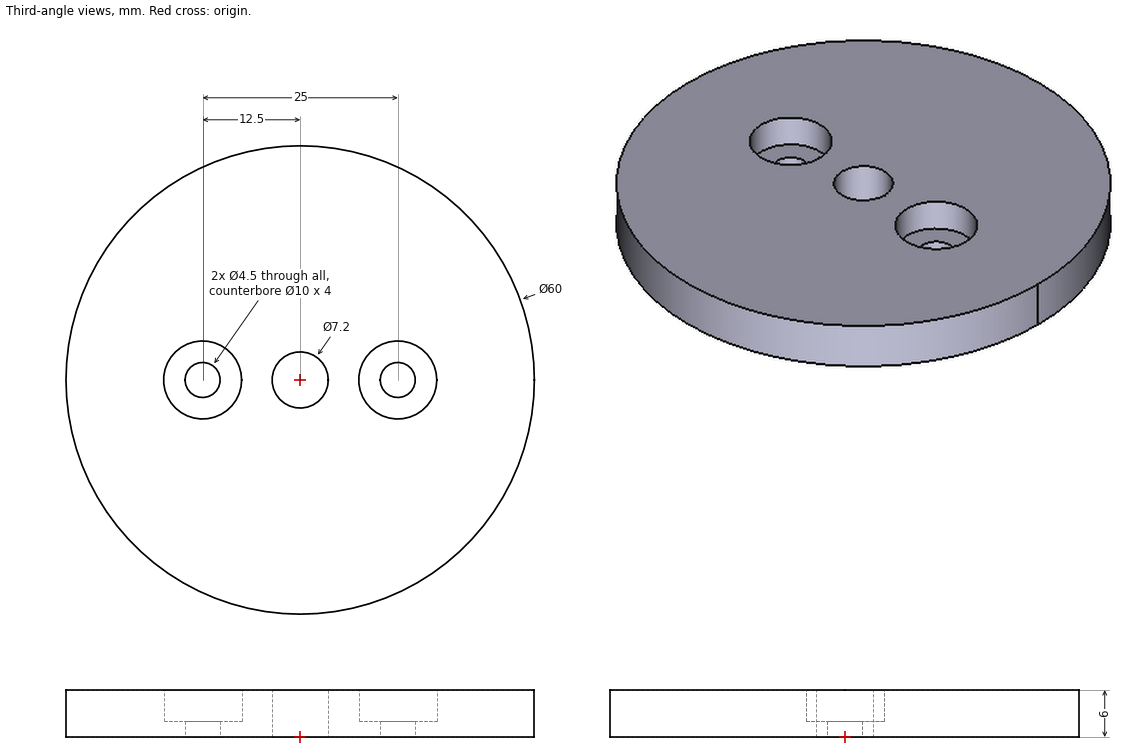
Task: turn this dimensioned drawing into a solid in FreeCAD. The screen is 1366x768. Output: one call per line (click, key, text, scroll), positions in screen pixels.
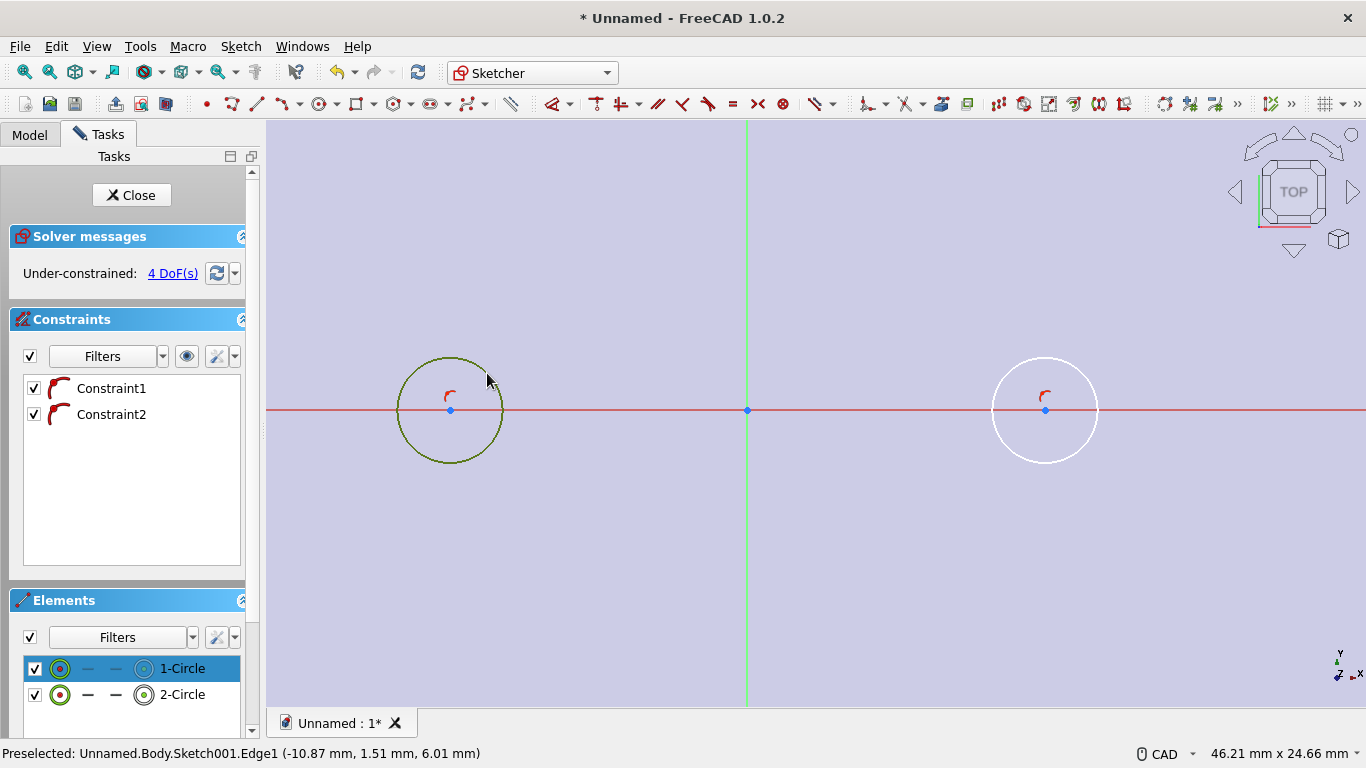
click(1082, 373)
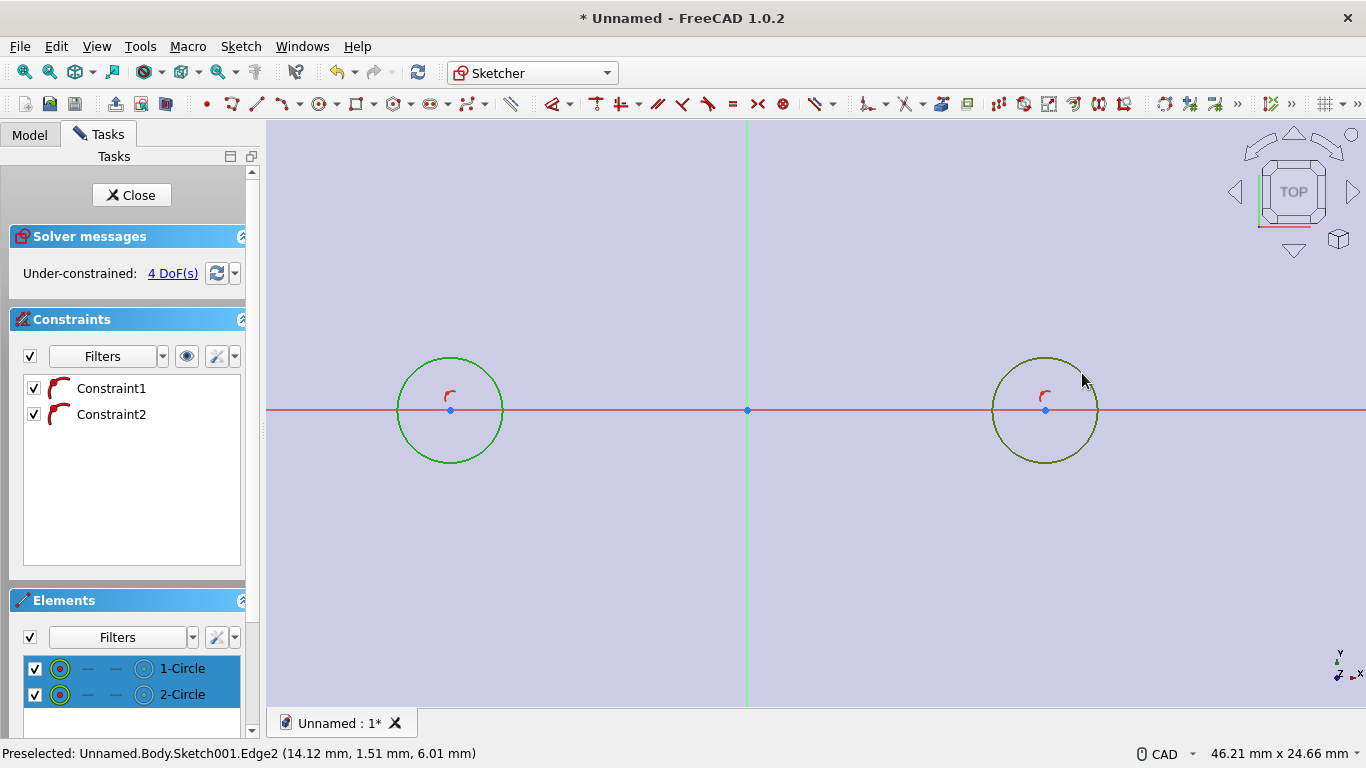
key(e)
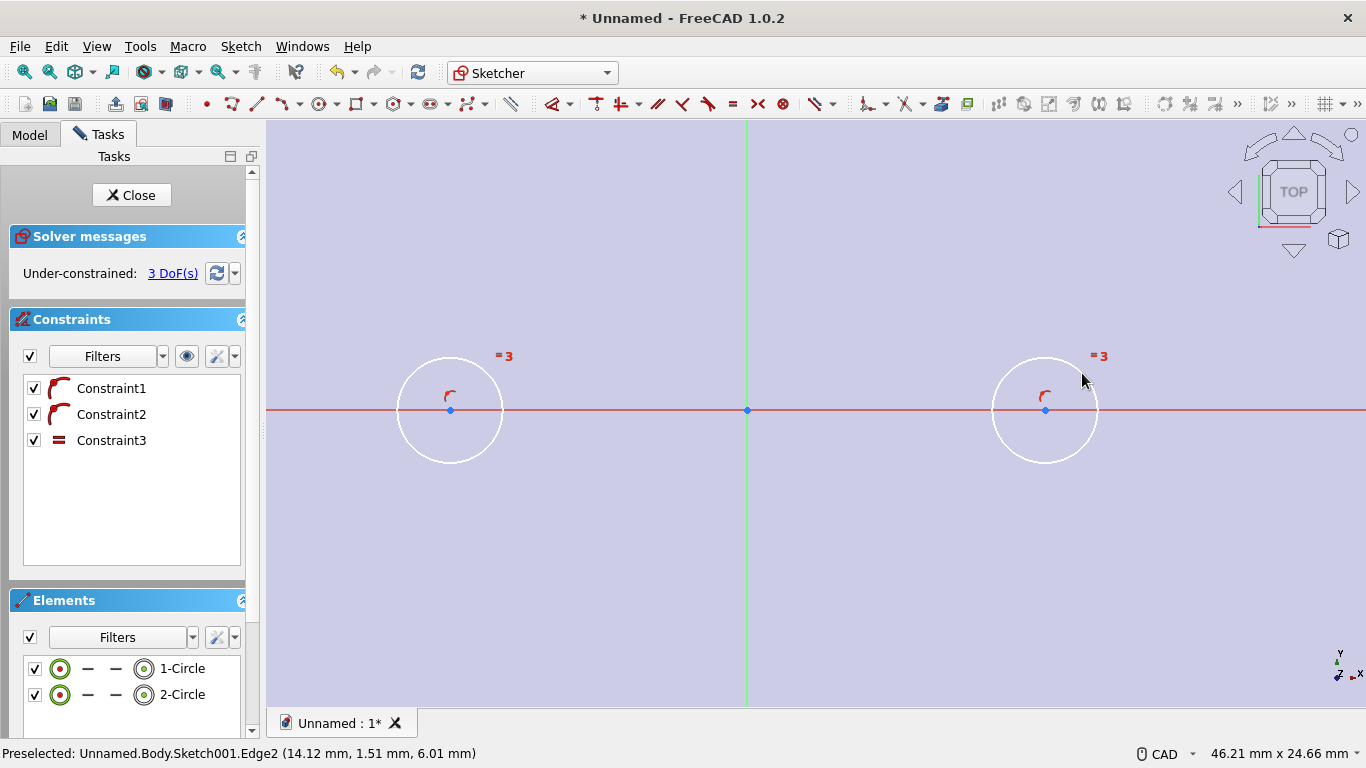
key(d)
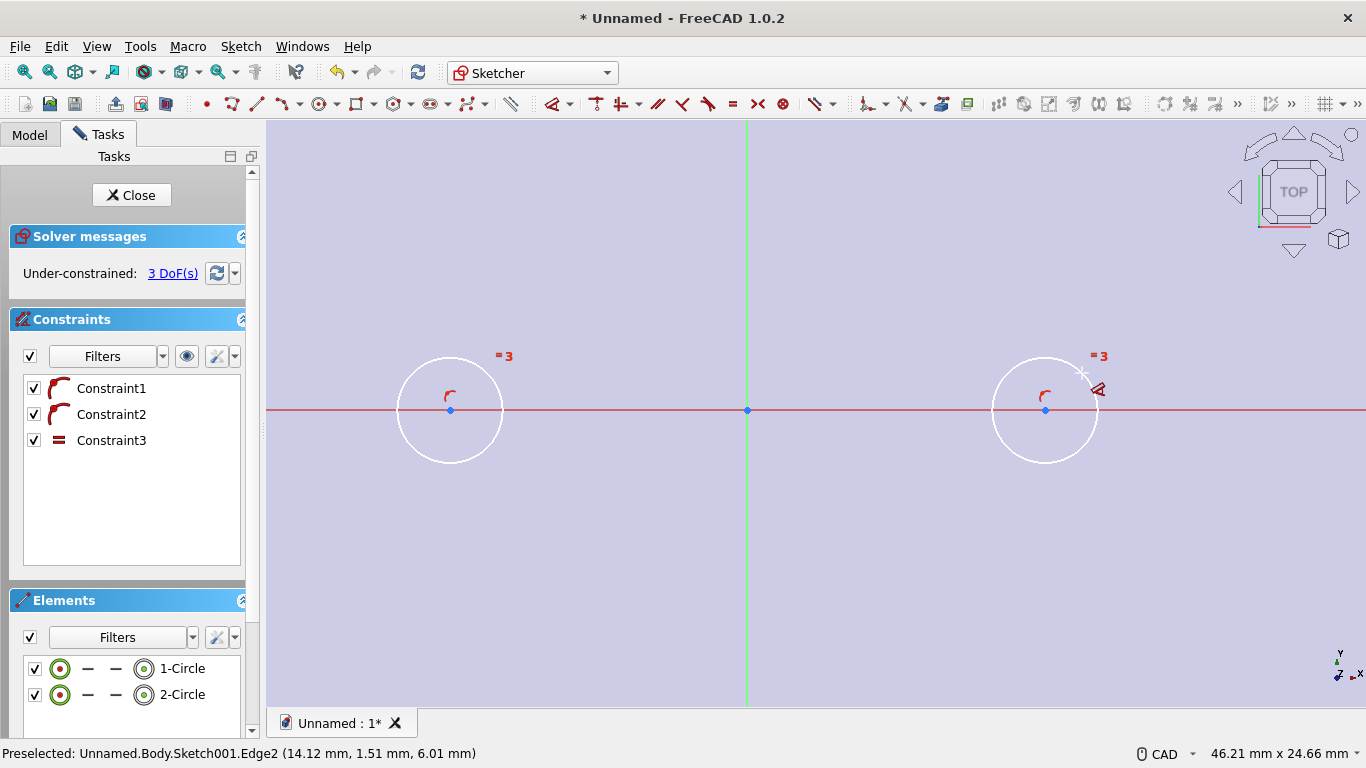
click(487, 373)
click(509, 350)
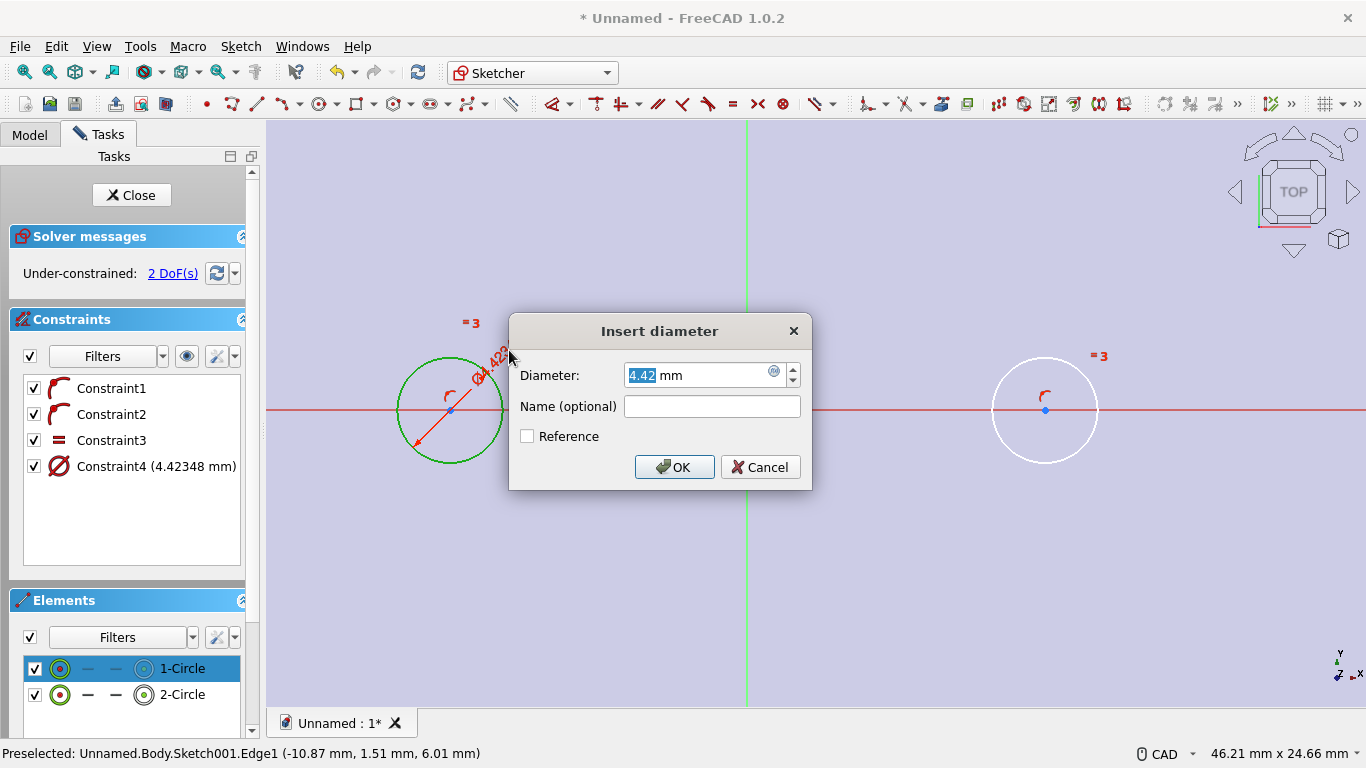
text(4.5)
key(Return)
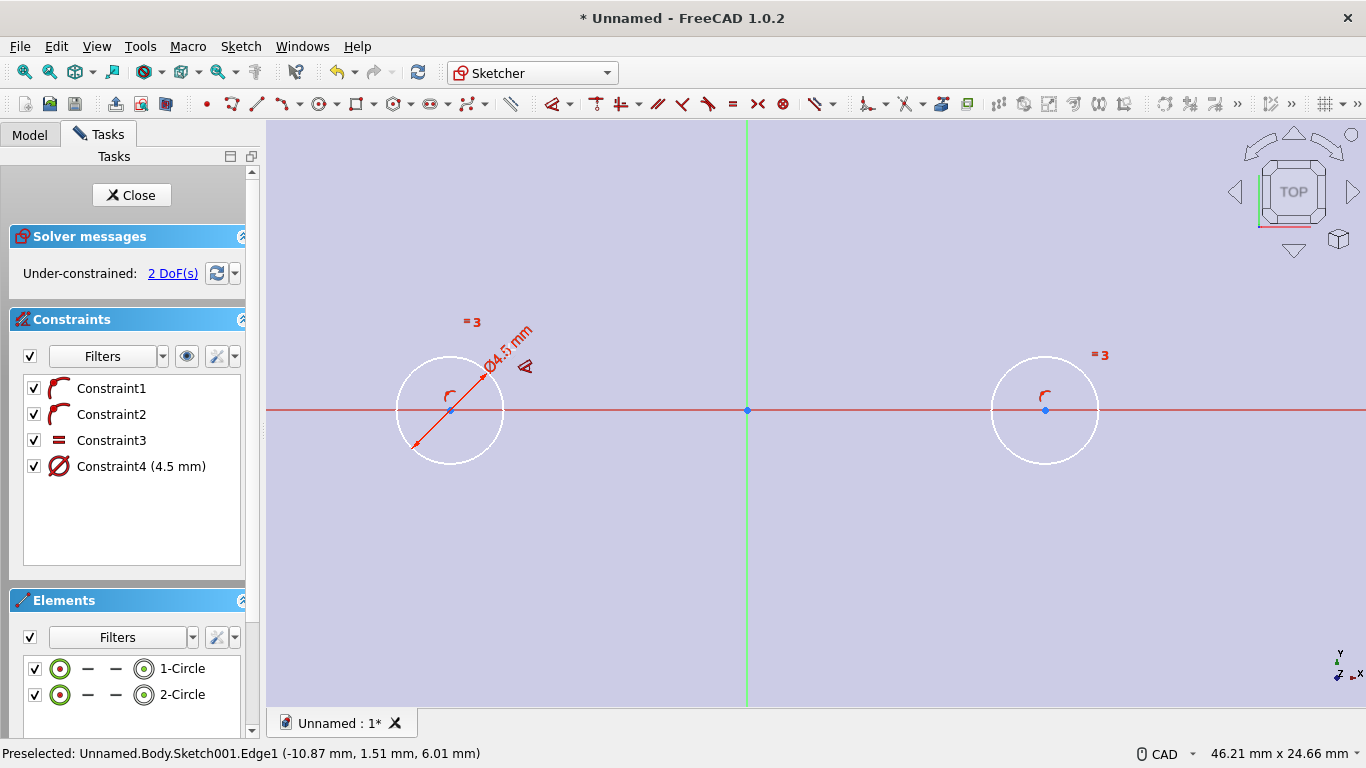
click(450, 410)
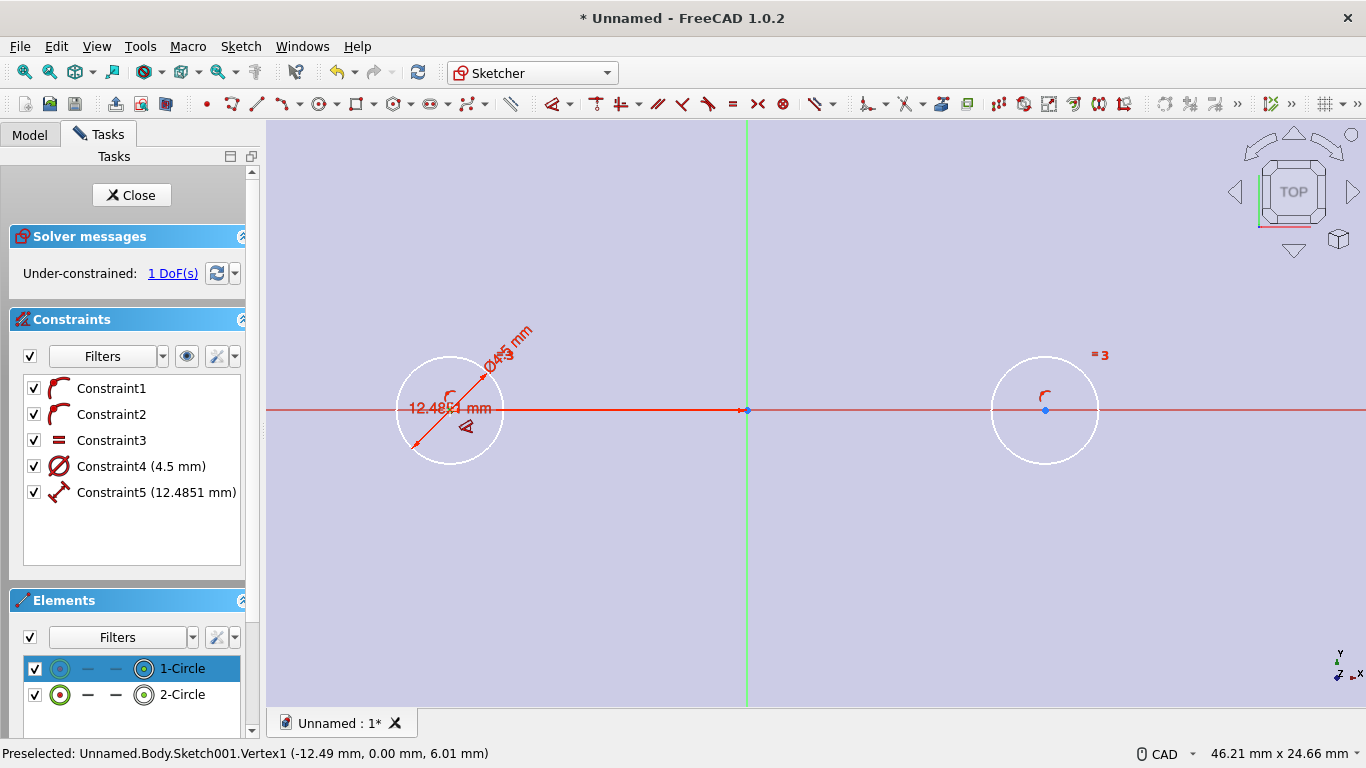
click(1045, 410)
click(611, 444)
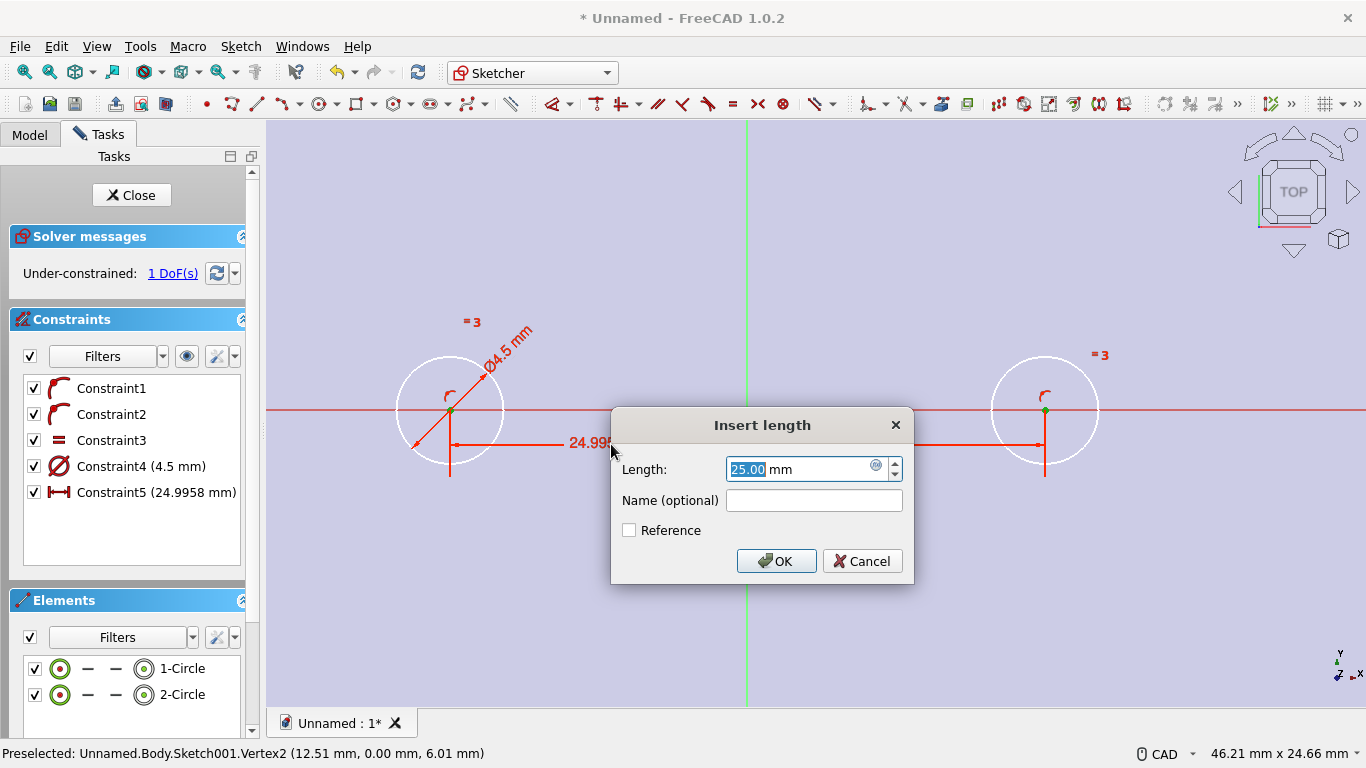
text(25)
key(Return)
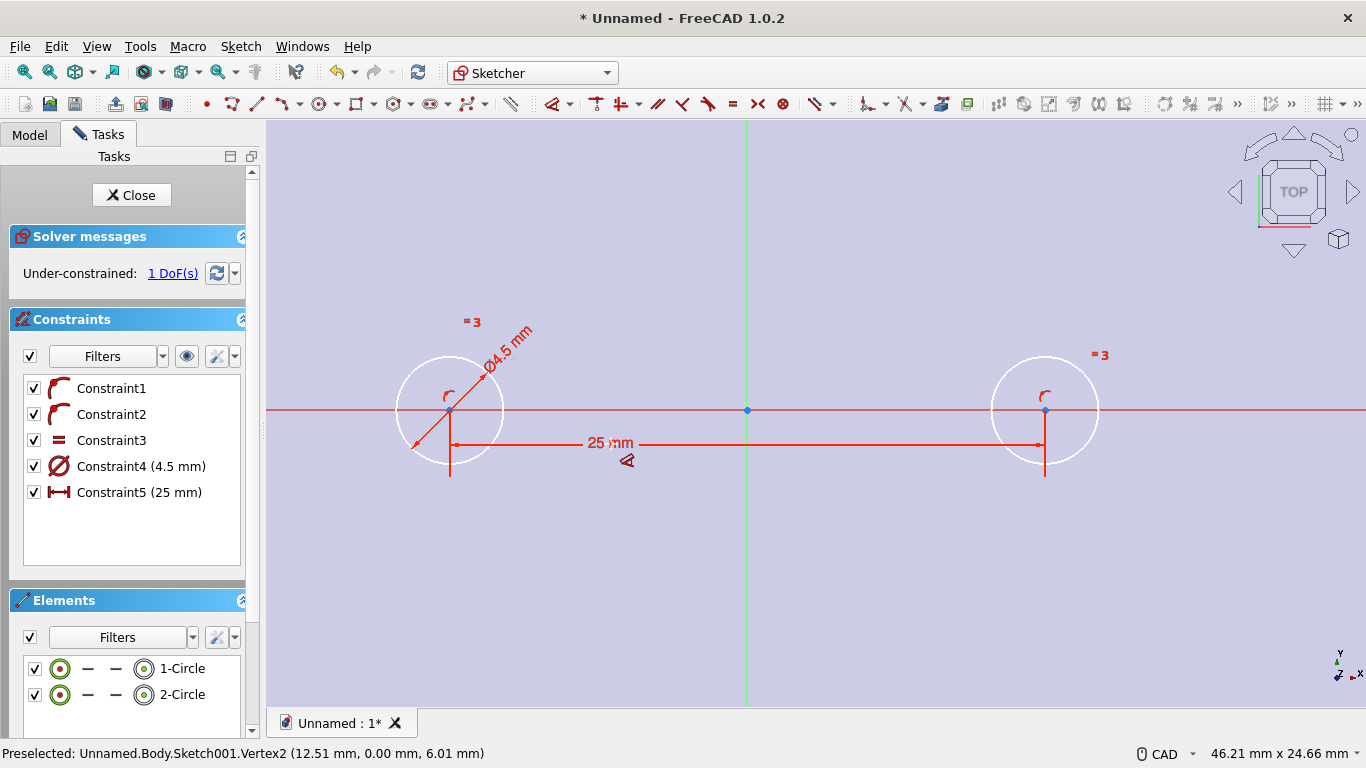
click(450, 410)
click(530, 444)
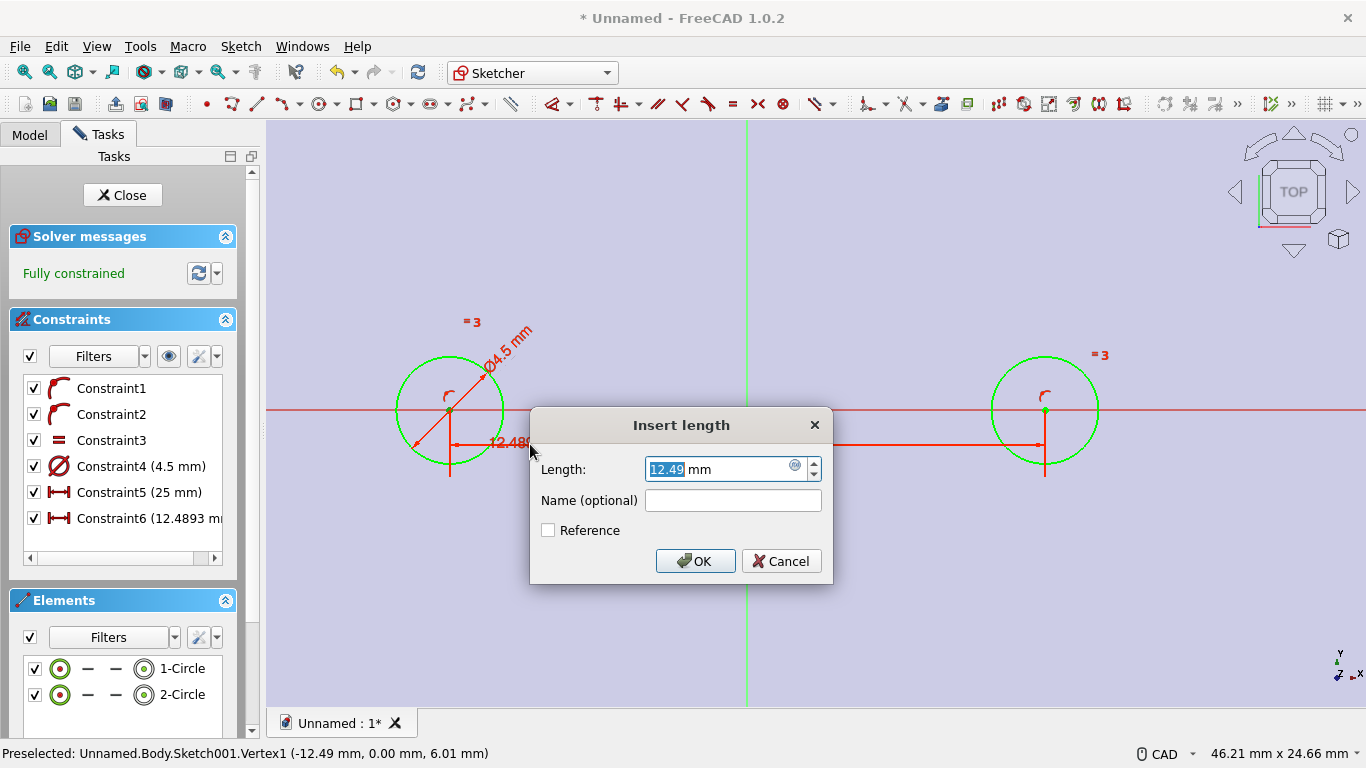
text(12.5)
key(Return)
key(Escape)